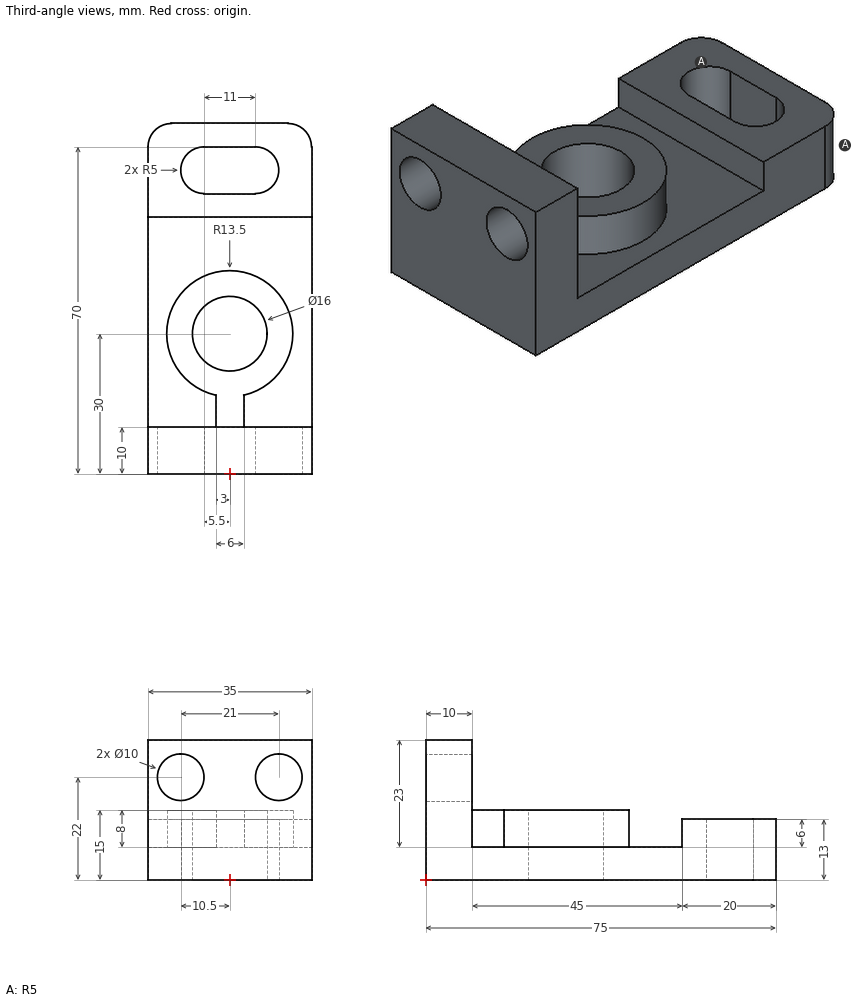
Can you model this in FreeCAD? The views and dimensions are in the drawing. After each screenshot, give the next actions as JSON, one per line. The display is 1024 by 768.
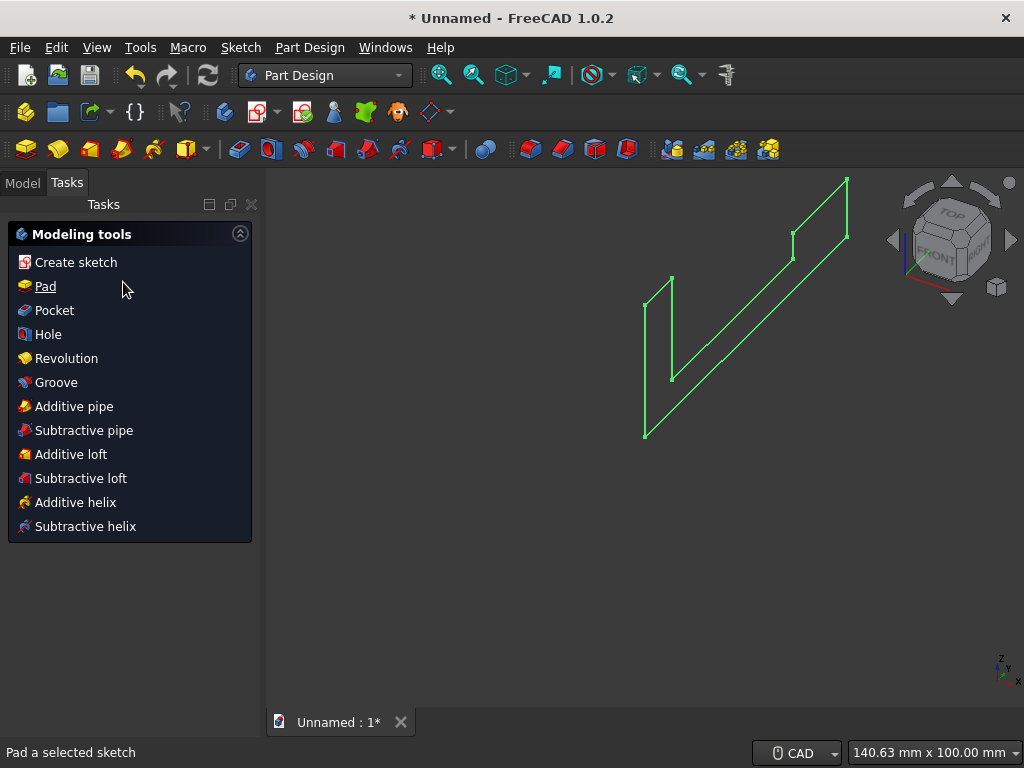
{"action": "left_click", "coordinate": [26, 150]}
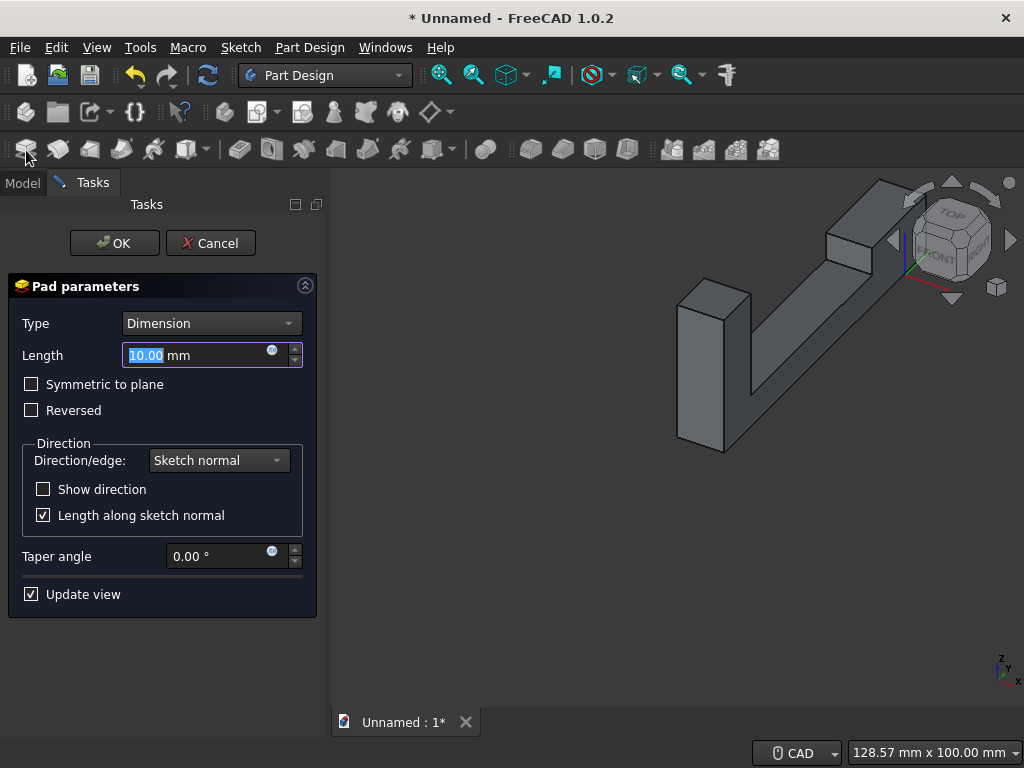
{"action": "type", "text": "35"}
{"action": "key", "text": "Tab"}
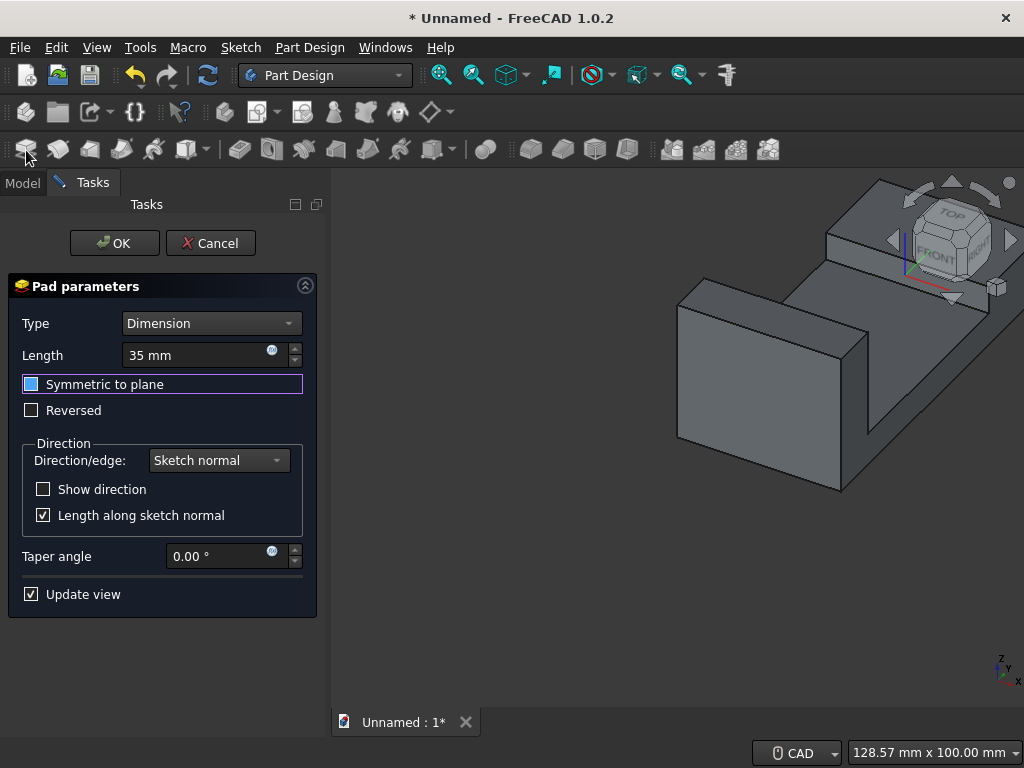
{"action": "left_click", "coordinate": [30, 384]}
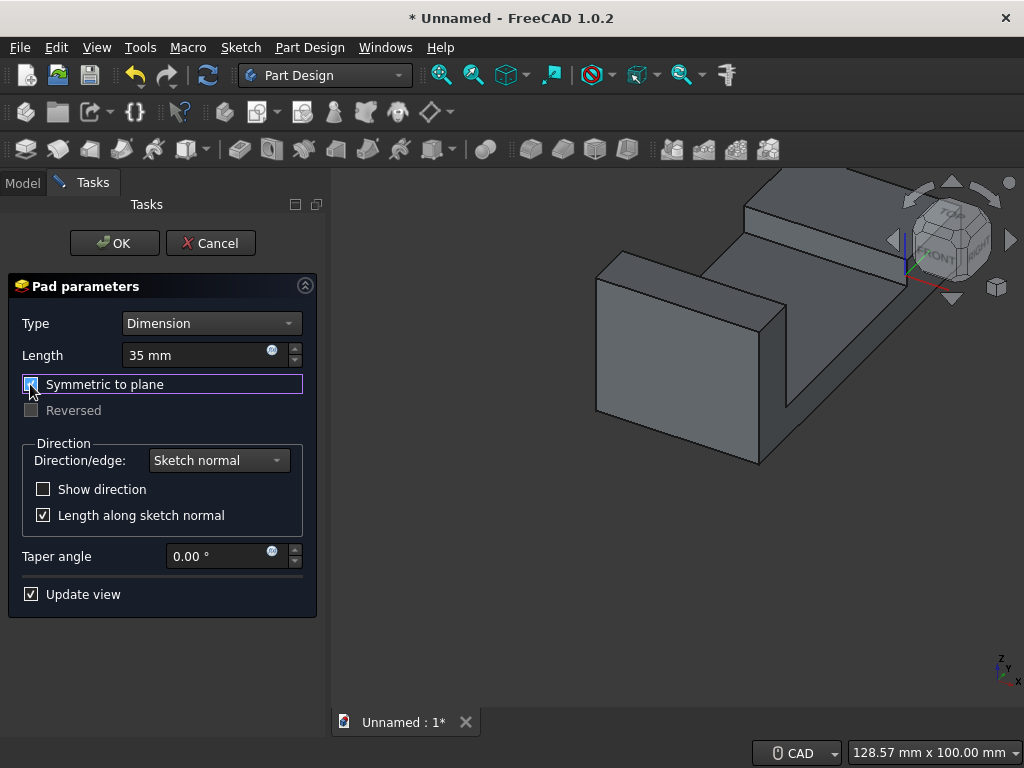
{"action": "left_click", "coordinate": [115, 243]}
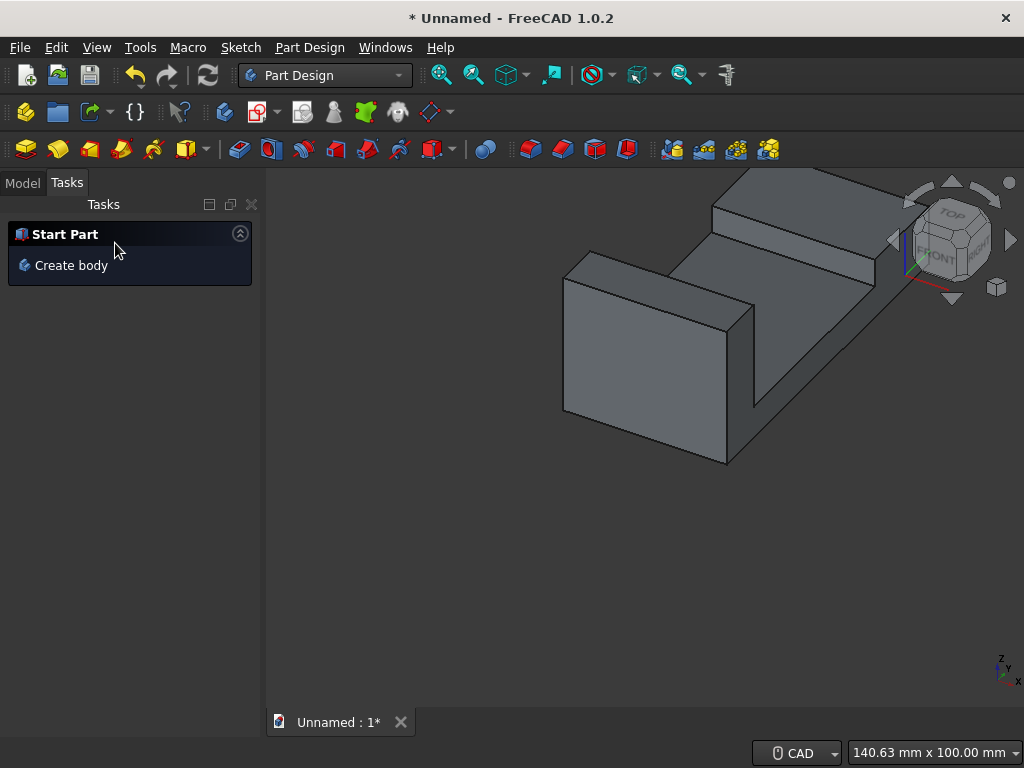
{"action": "left_click", "coordinate": [442, 76]}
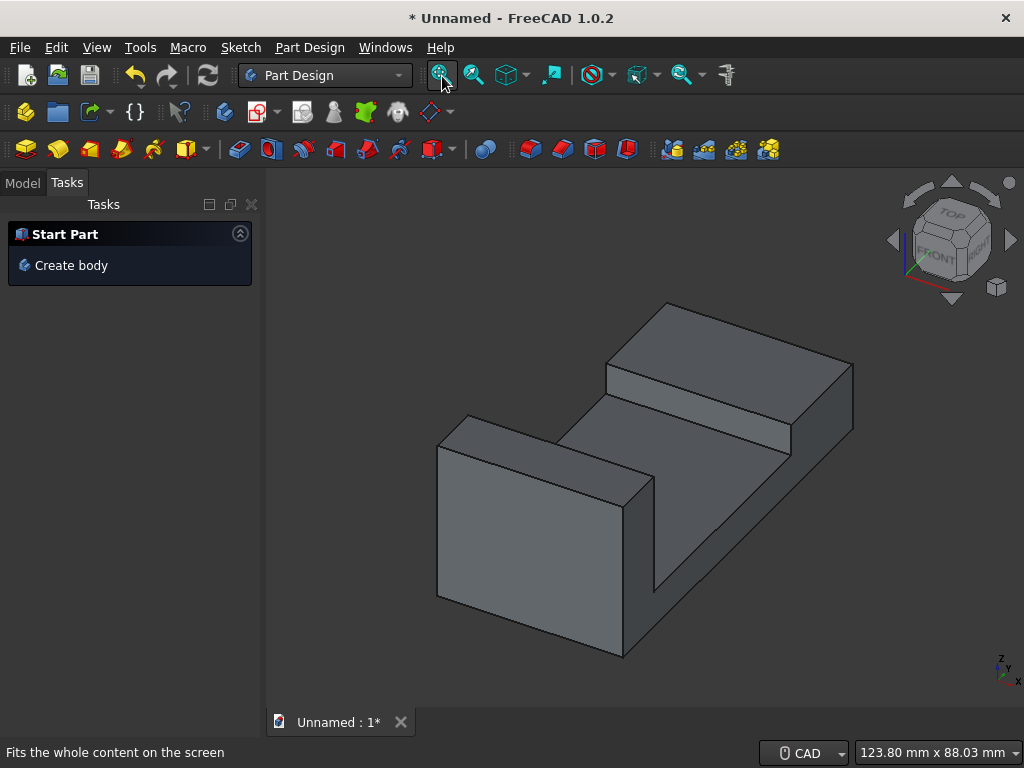
{"action": "key", "text": "0"}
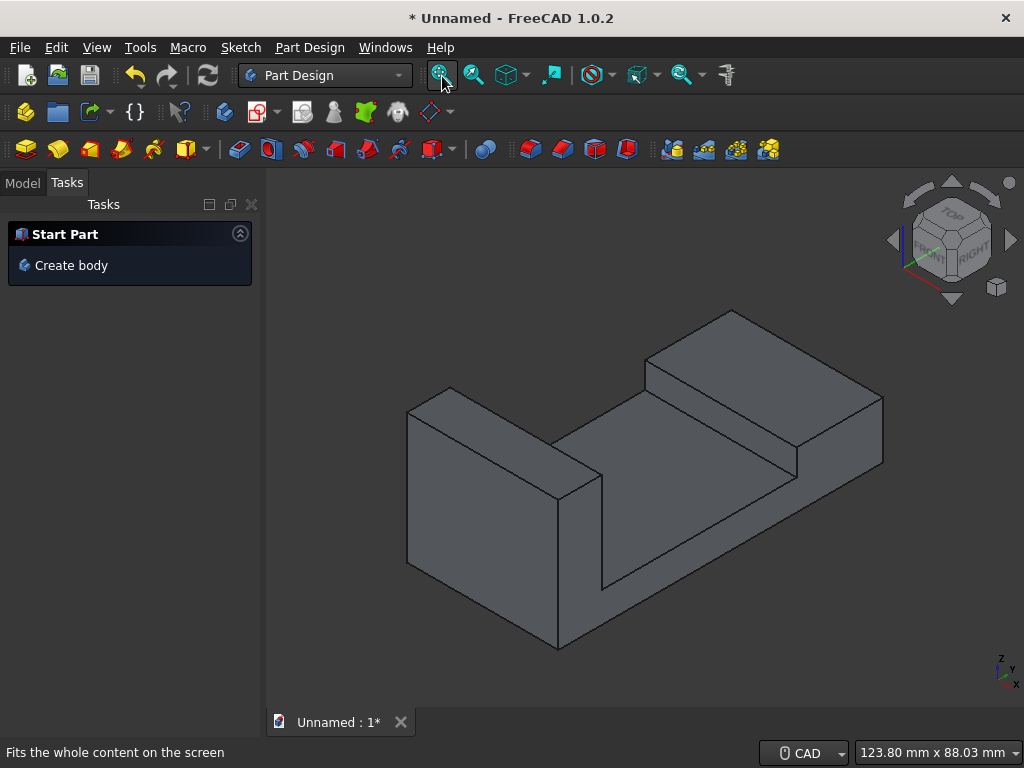
{"action": "key", "text": "2"}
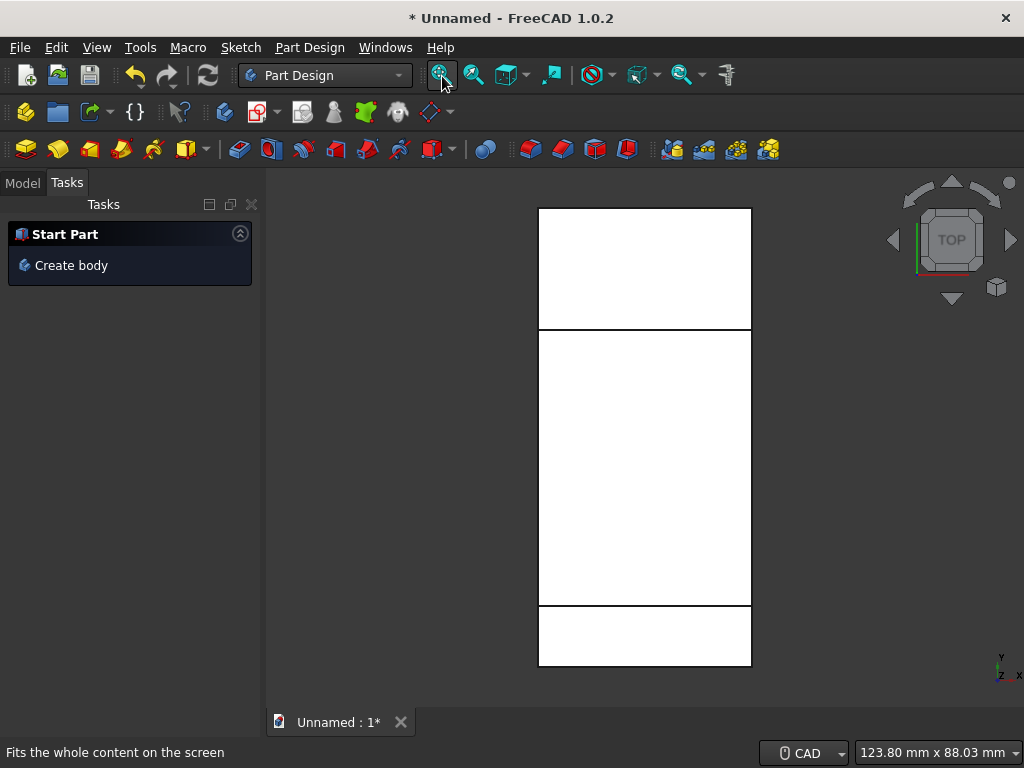
{"action": "key", "text": "1"}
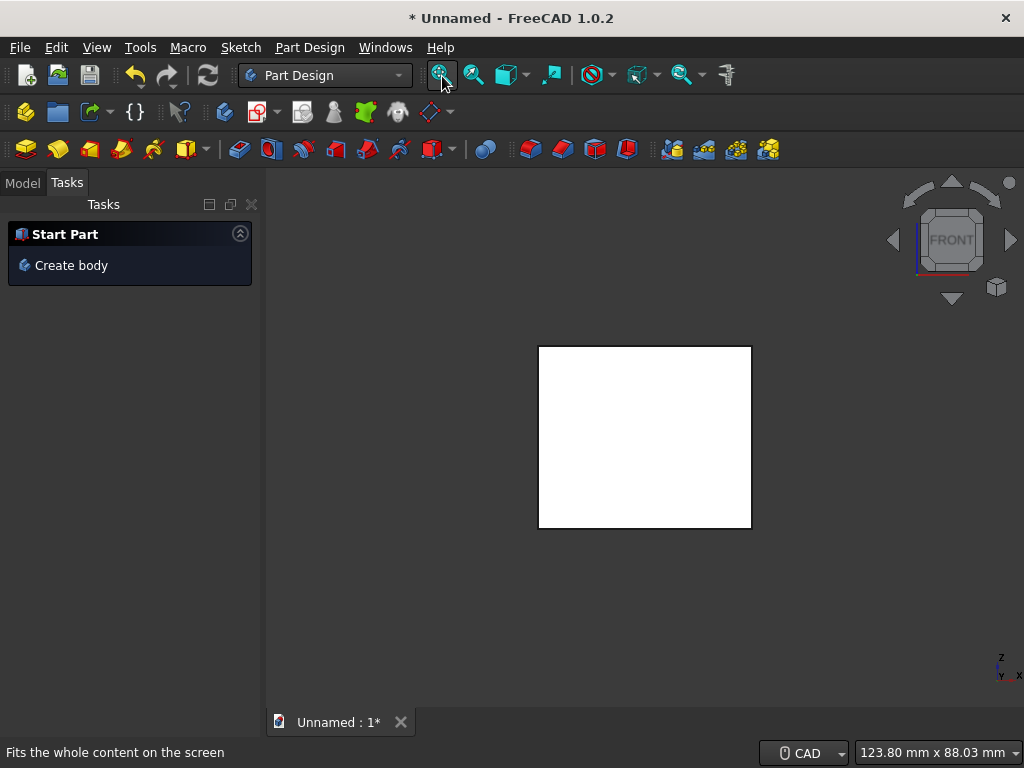
{"action": "key", "text": "v f"}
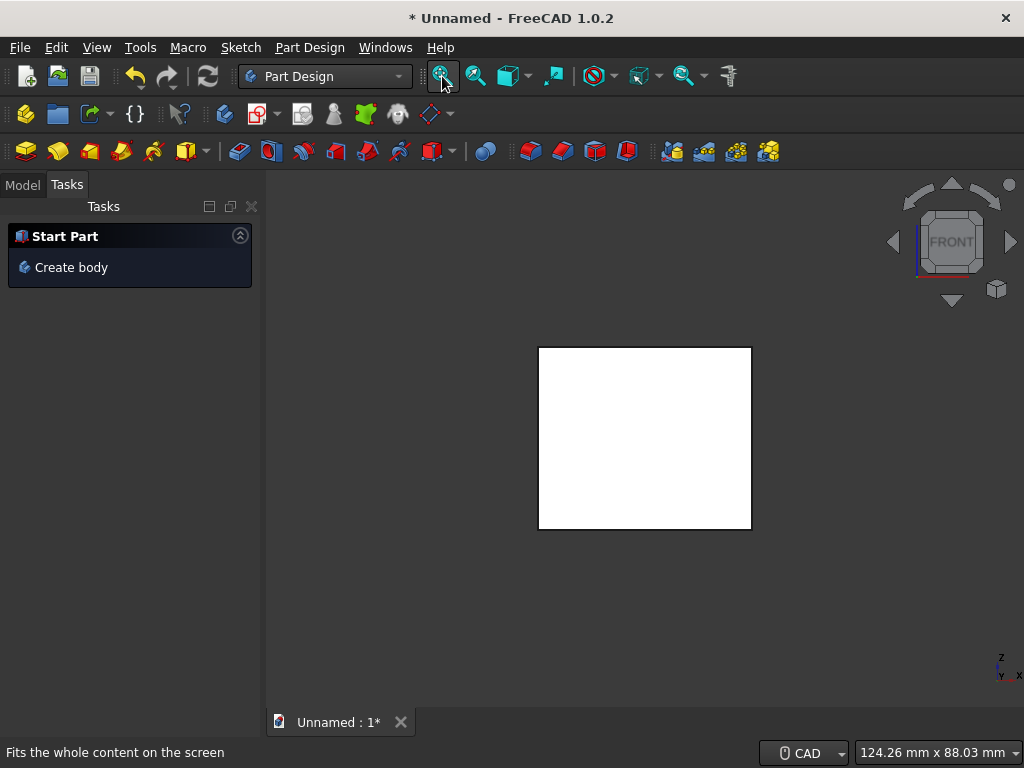
{"action": "key", "text": "3"}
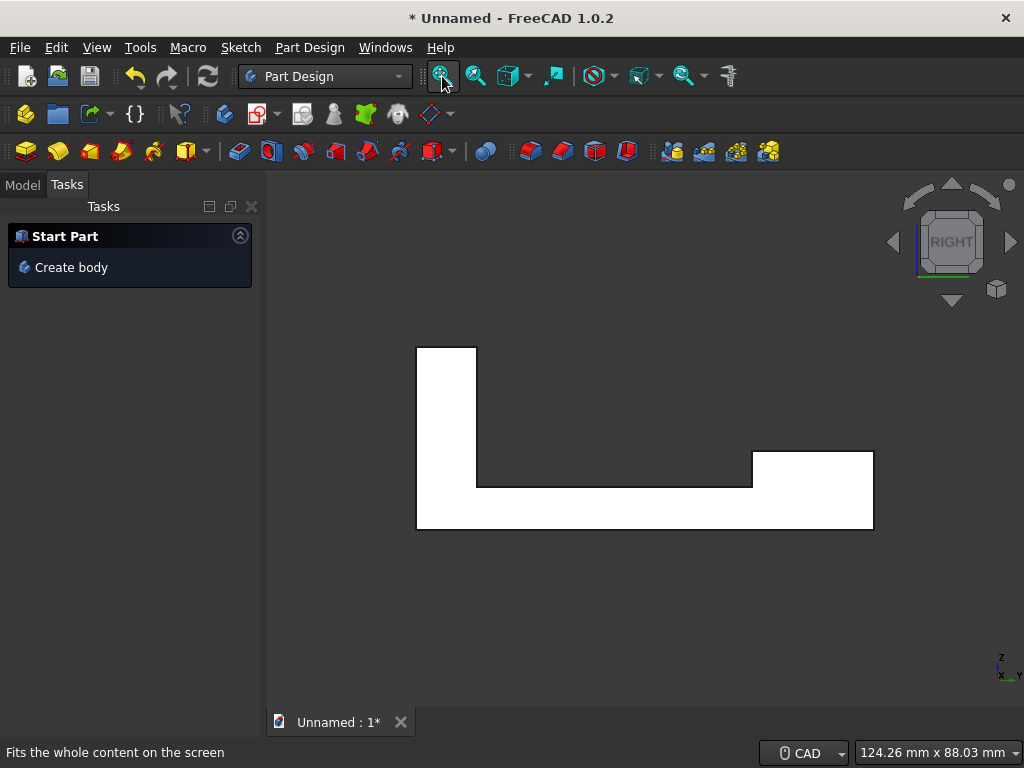
{"action": "left_click", "coordinate": [874, 489]}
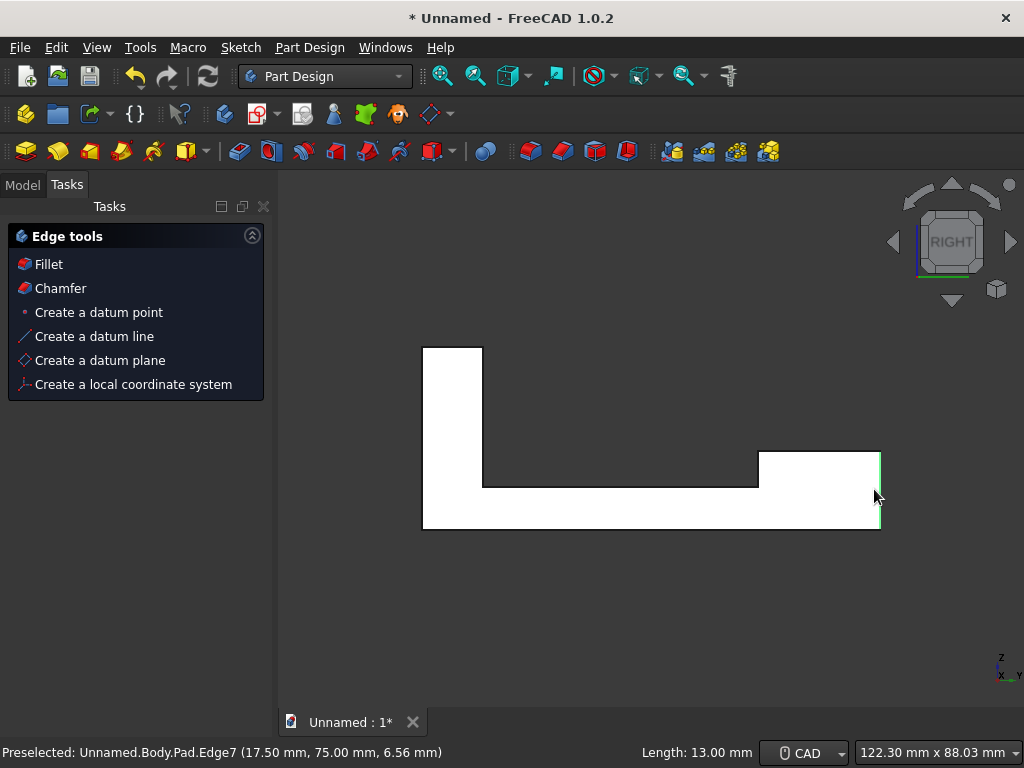
{"action": "key", "text": "5"}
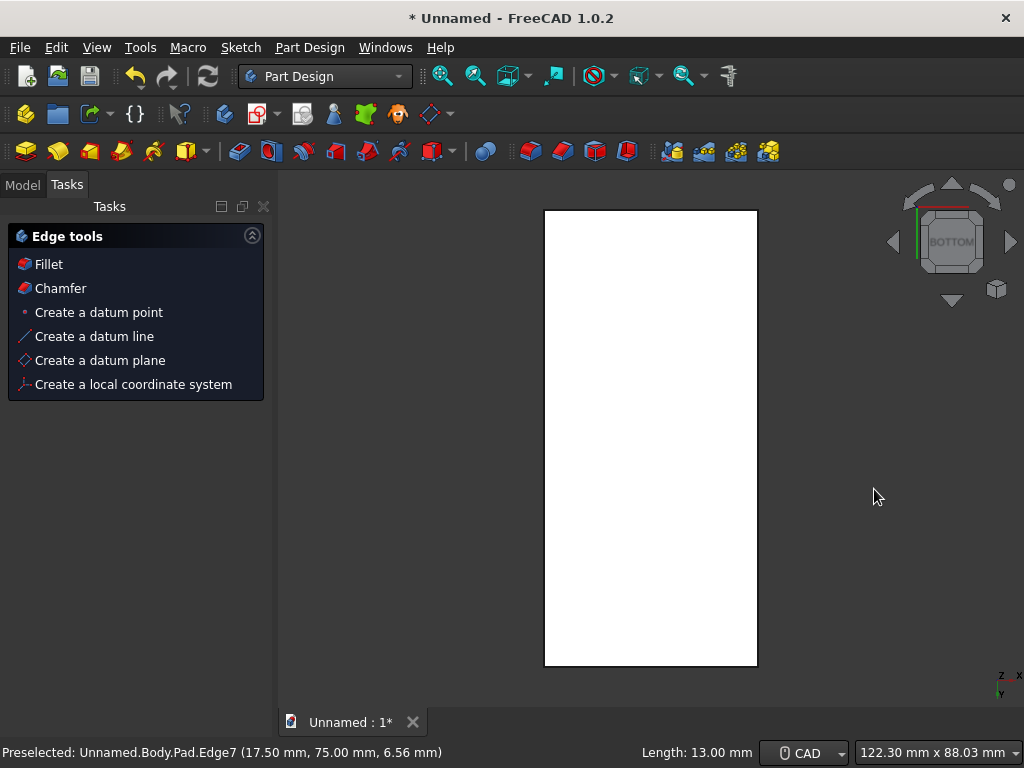
{"action": "key", "text": "4"}